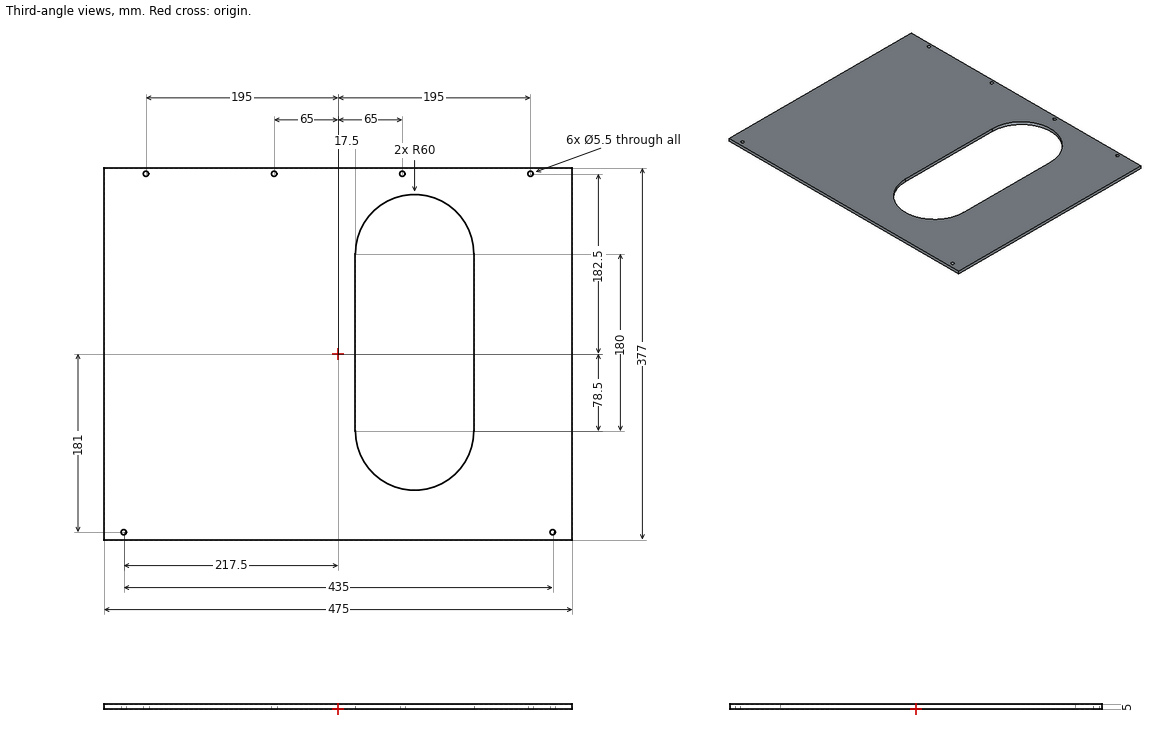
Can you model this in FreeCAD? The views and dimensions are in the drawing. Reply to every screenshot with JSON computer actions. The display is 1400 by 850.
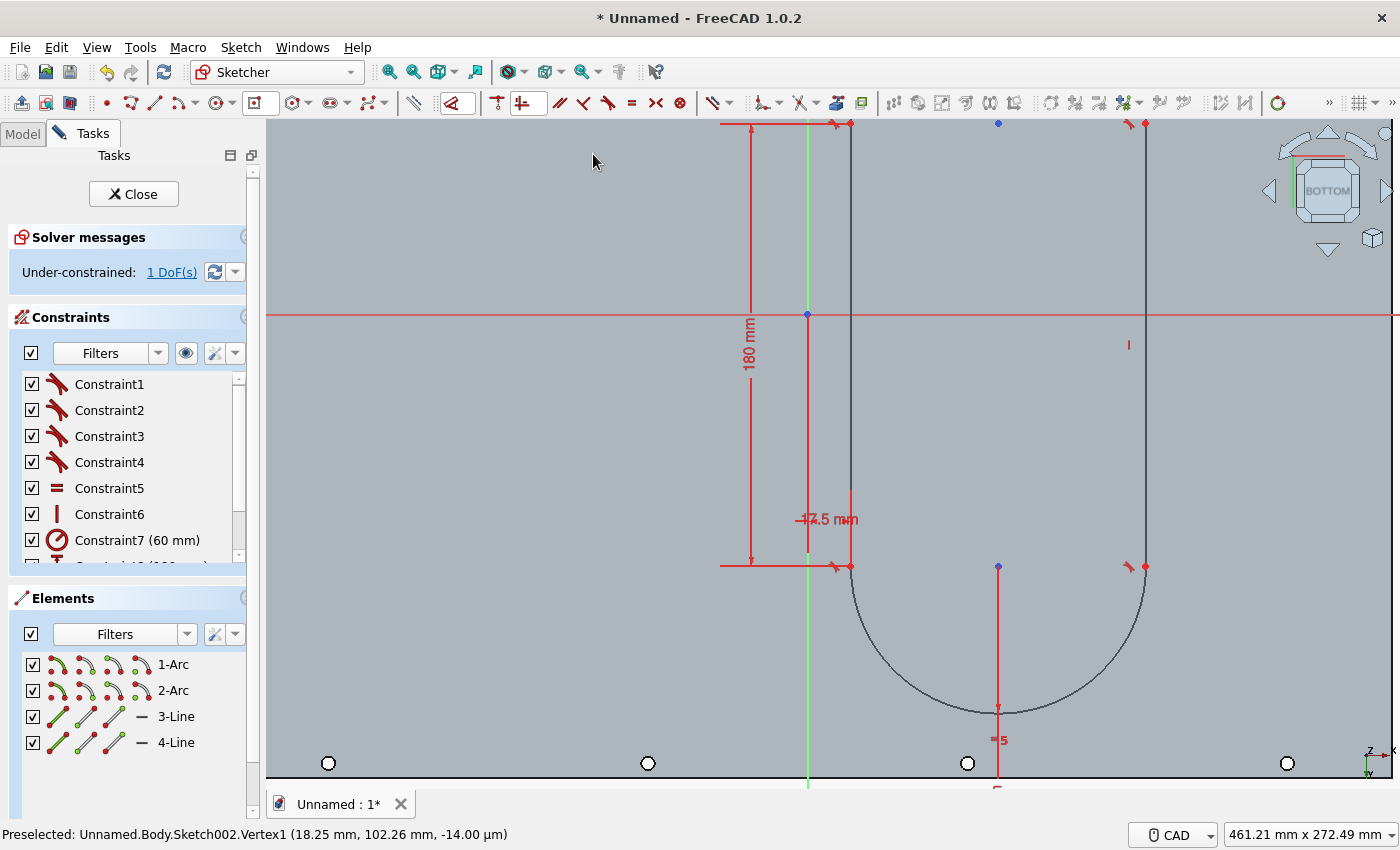
{"action": "scroll", "coordinate": [506, 589], "scroll_direction": "down", "scroll_amount": 3}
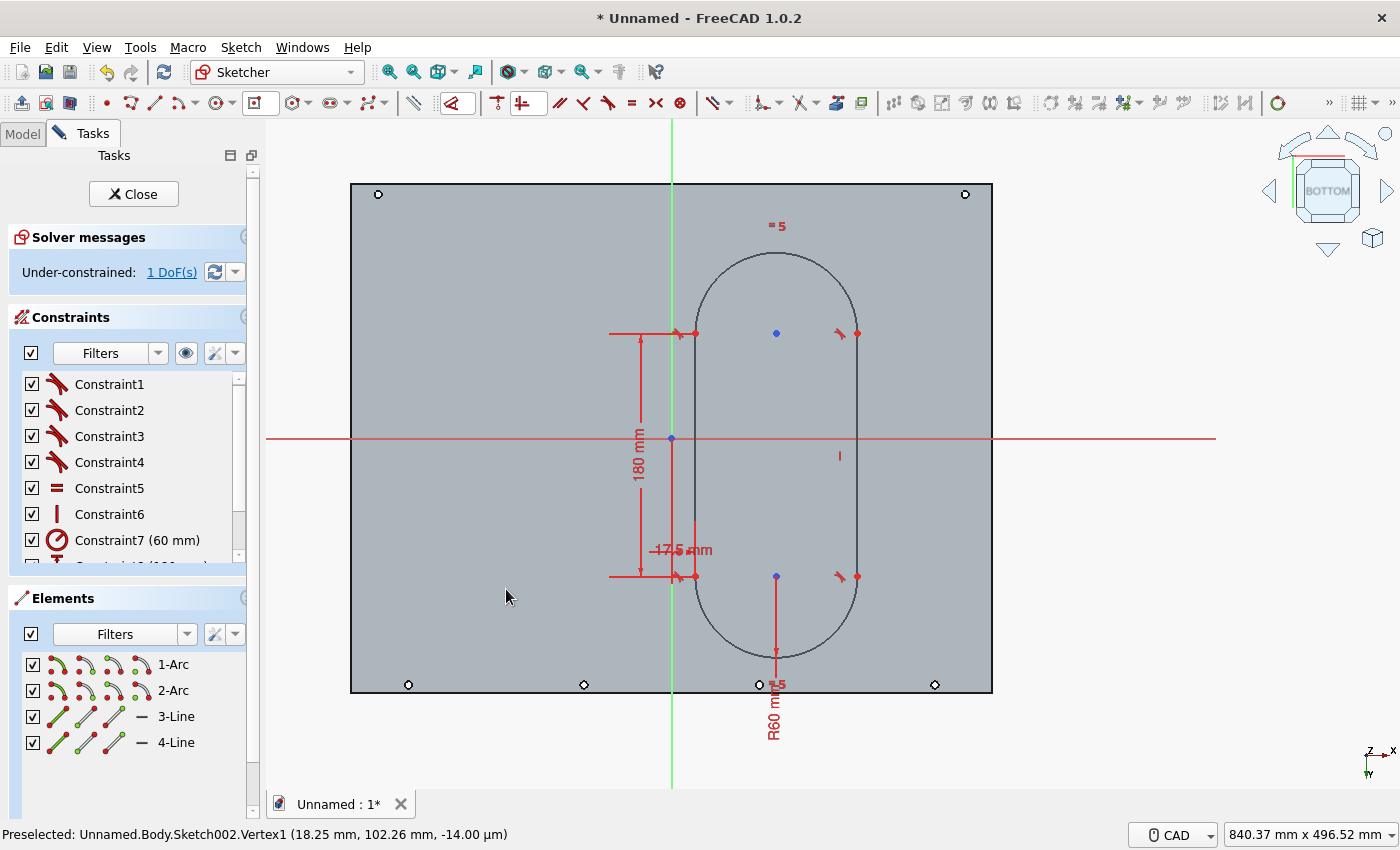
{"action": "left_click", "coordinate": [857, 334]}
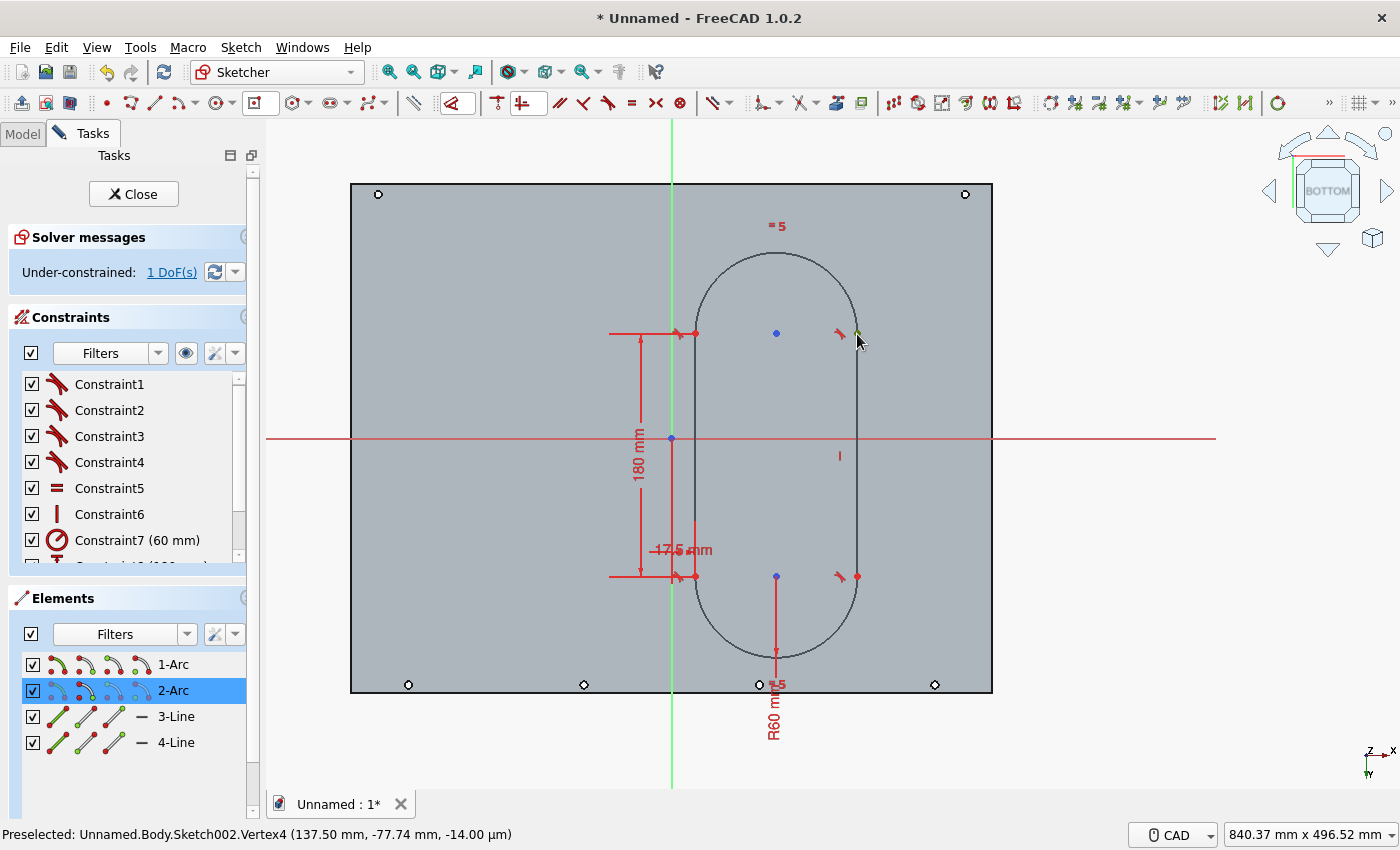
{"action": "key", "text": "i"}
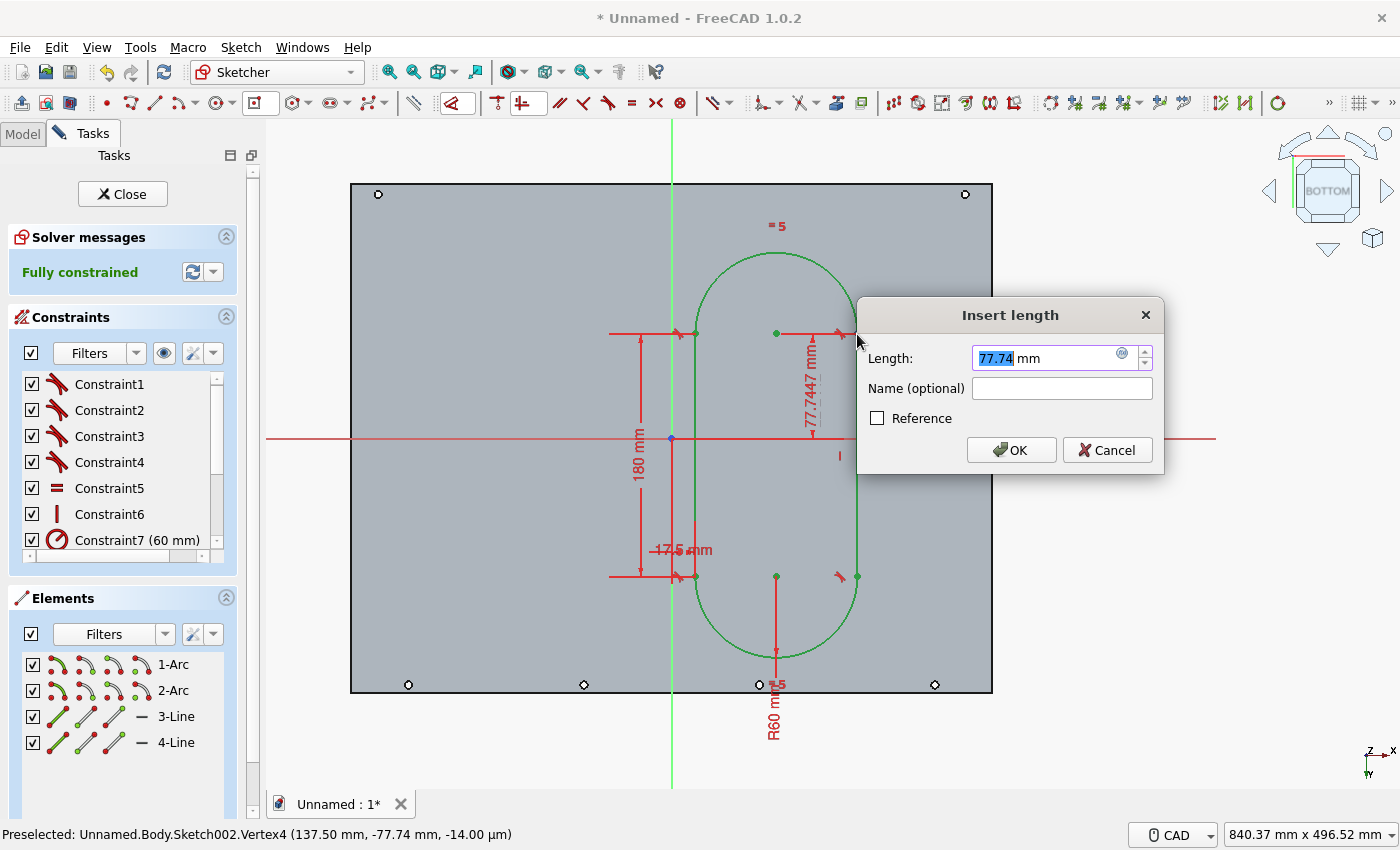
{"action": "type", "text": "78.5"}
{"action": "key", "text": "Return"}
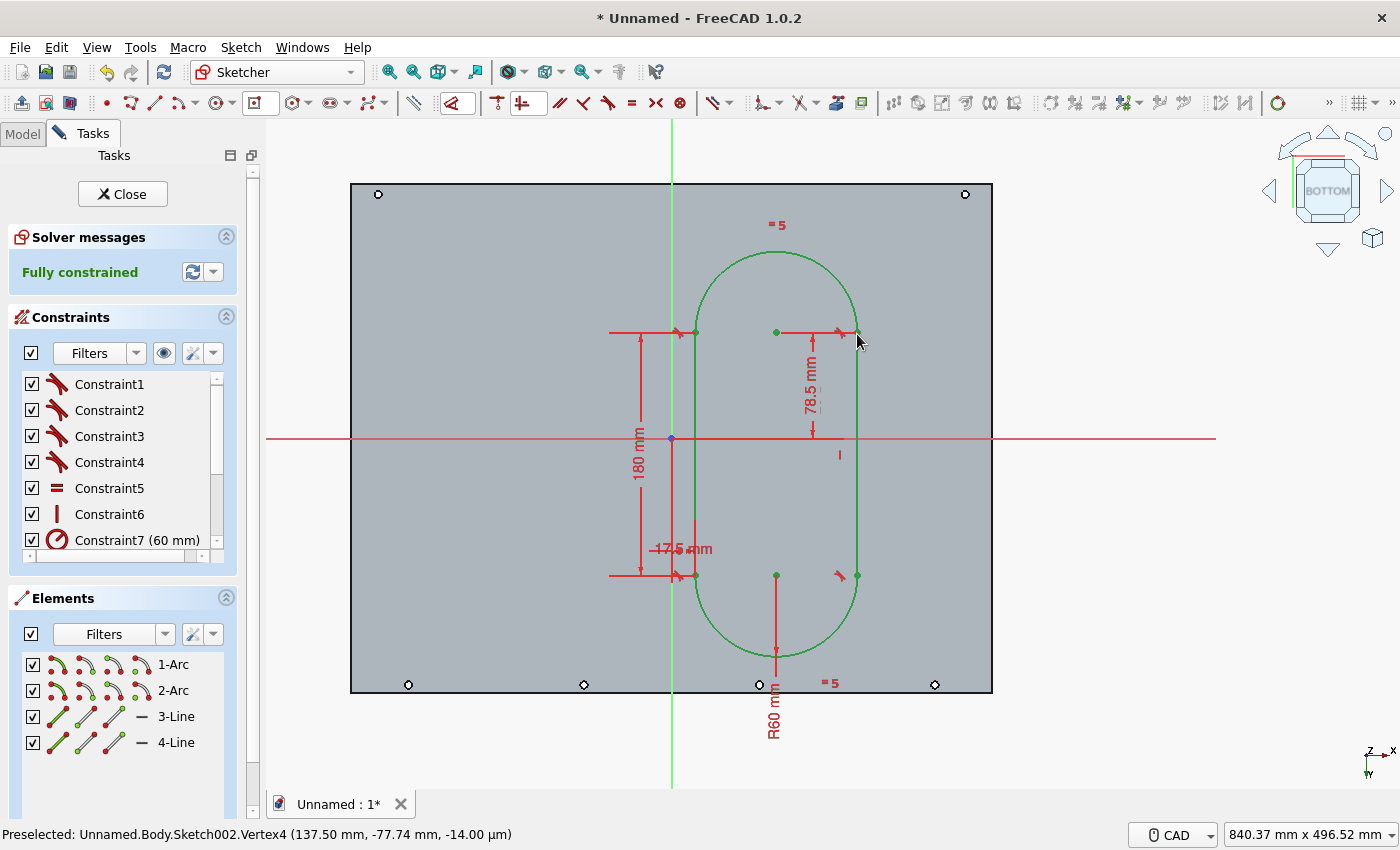
{"action": "left_click", "coordinate": [123, 194]}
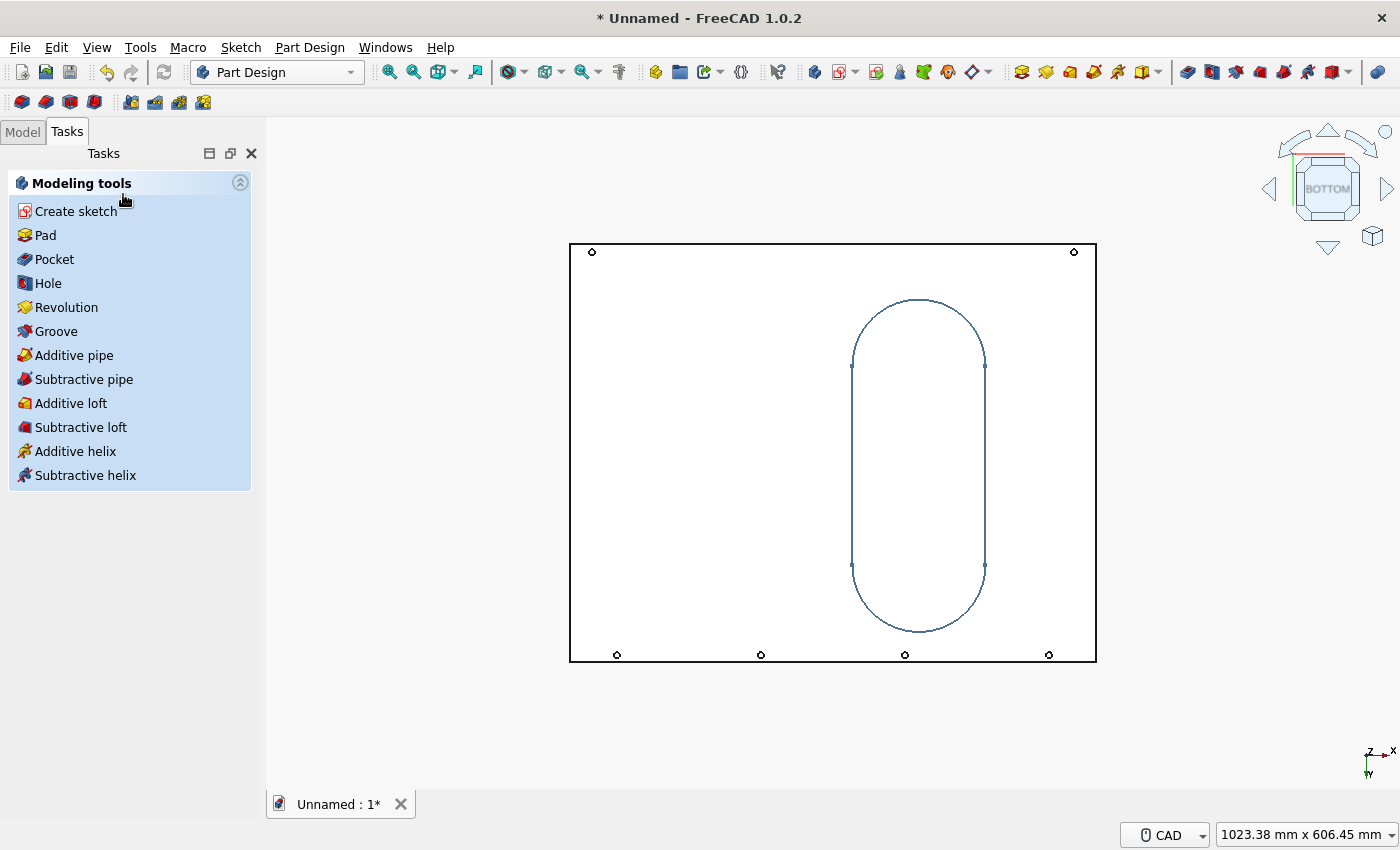
{"action": "left_click", "coordinate": [1188, 72]}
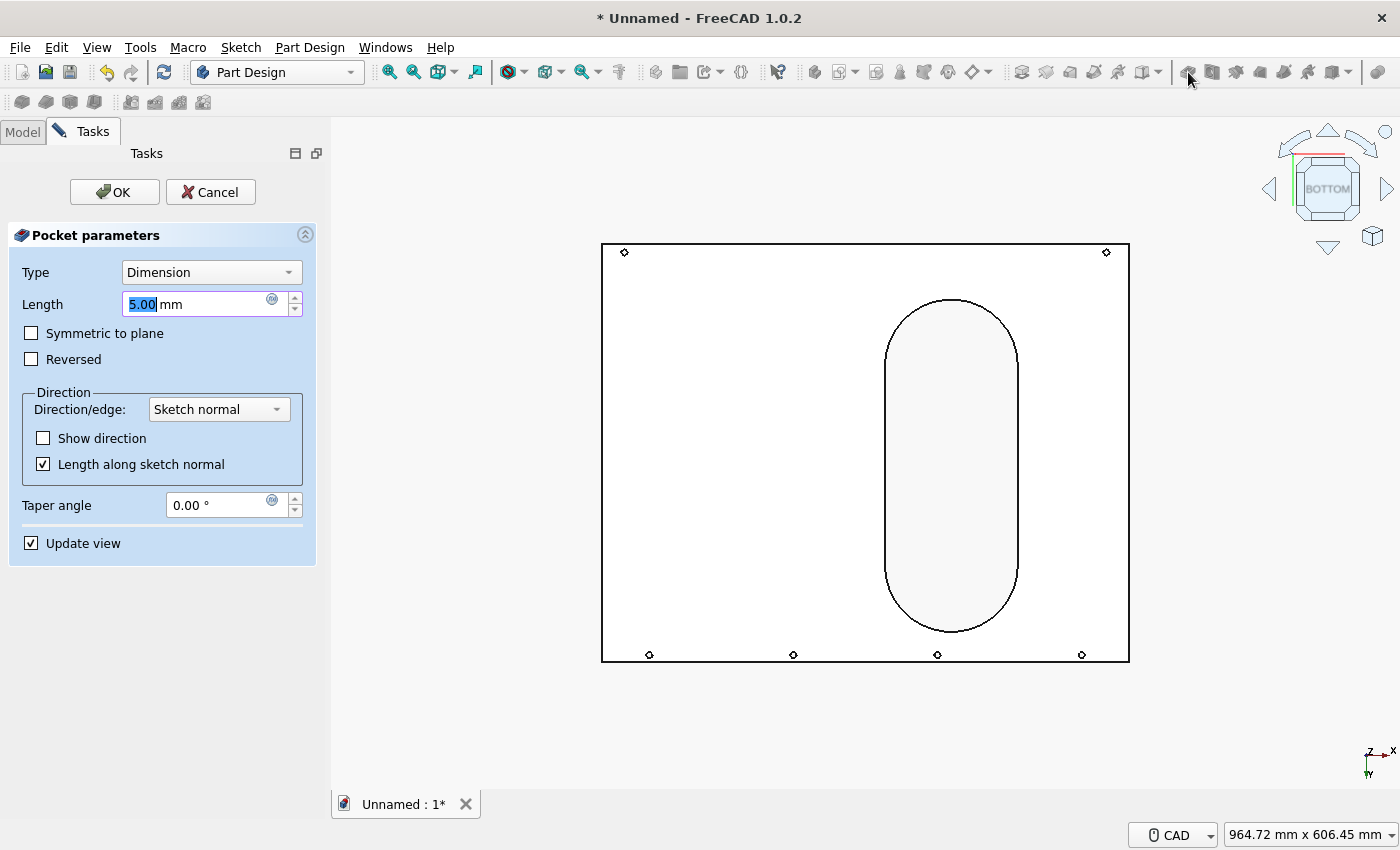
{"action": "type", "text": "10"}
{"action": "key", "text": "Tab"}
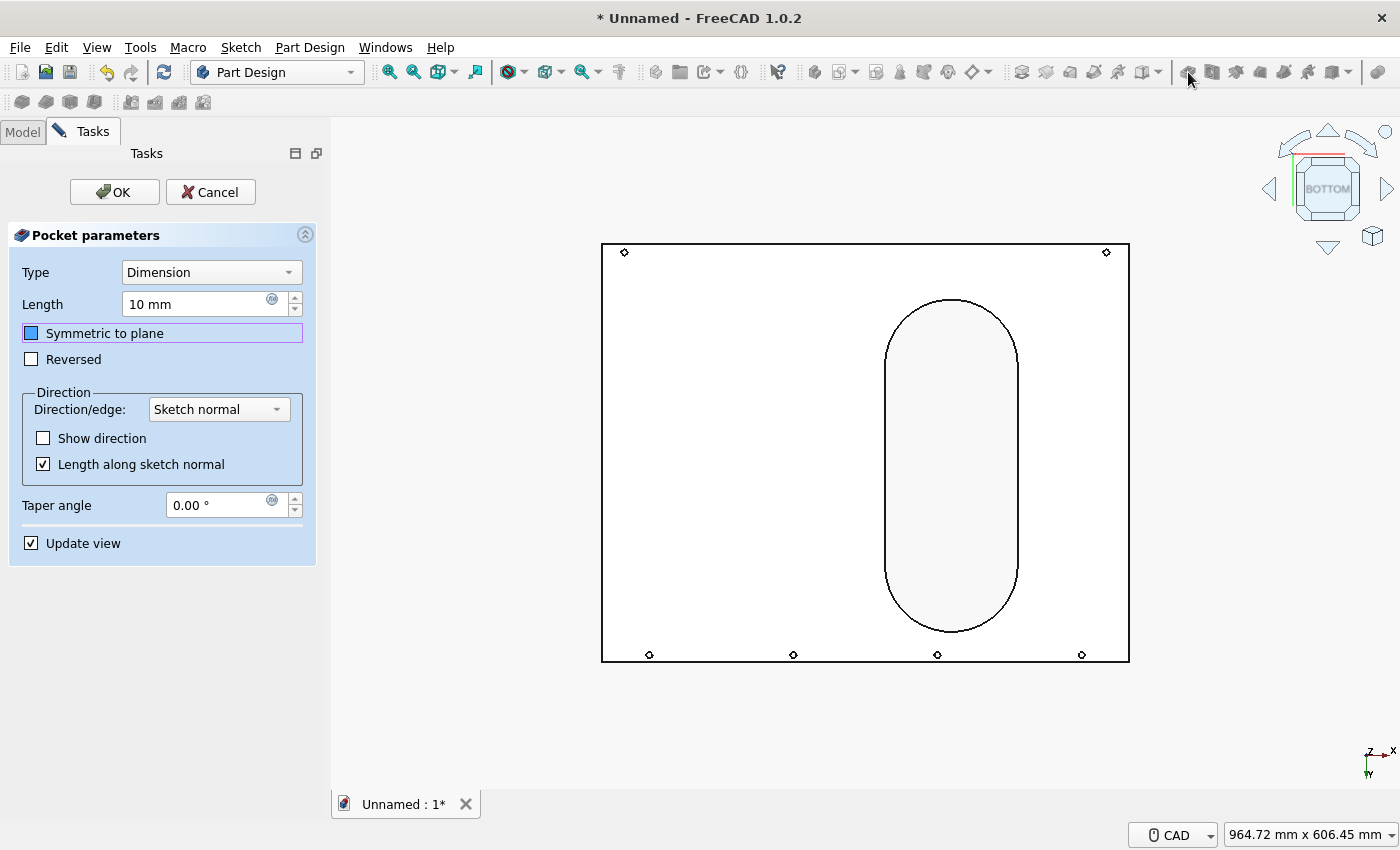
{"action": "left_click", "coordinate": [115, 192]}